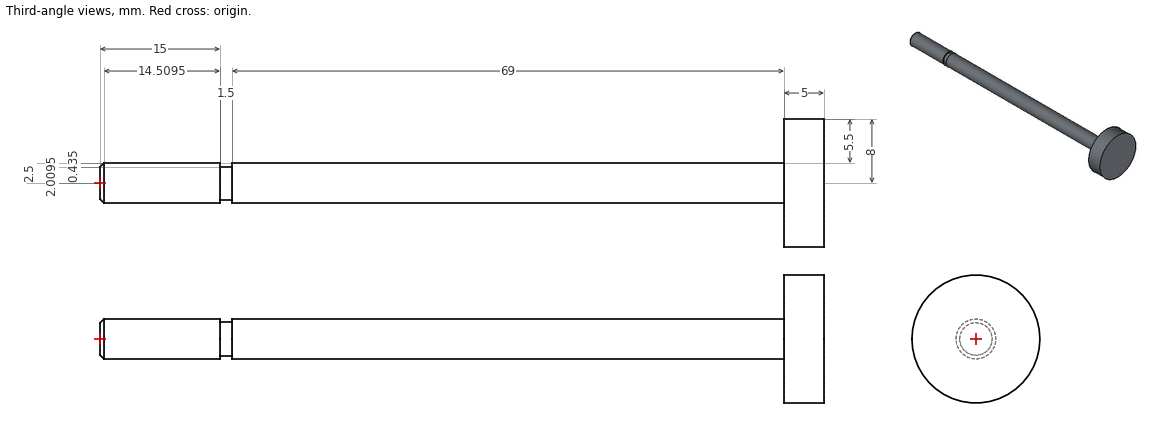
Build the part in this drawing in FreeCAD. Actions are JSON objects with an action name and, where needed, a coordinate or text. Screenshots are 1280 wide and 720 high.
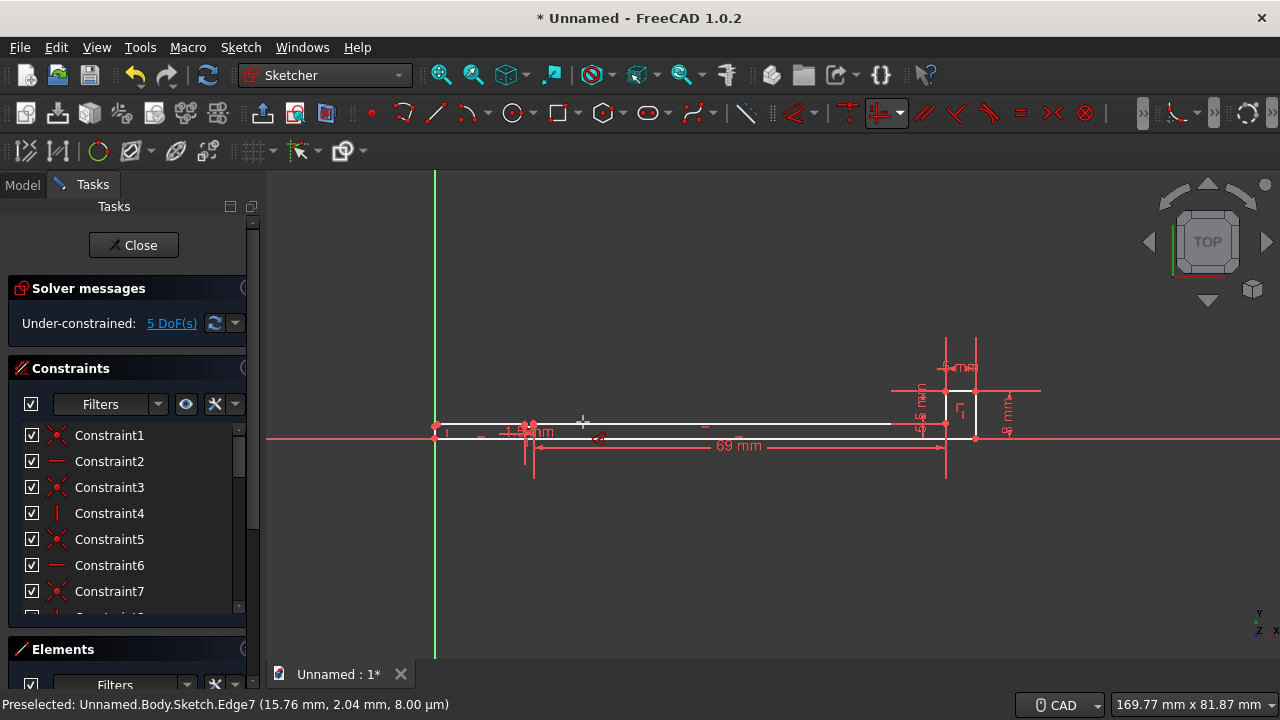
{"action": "scroll", "coordinate": [525, 427], "scroll_direction": "up", "scroll_amount": 8}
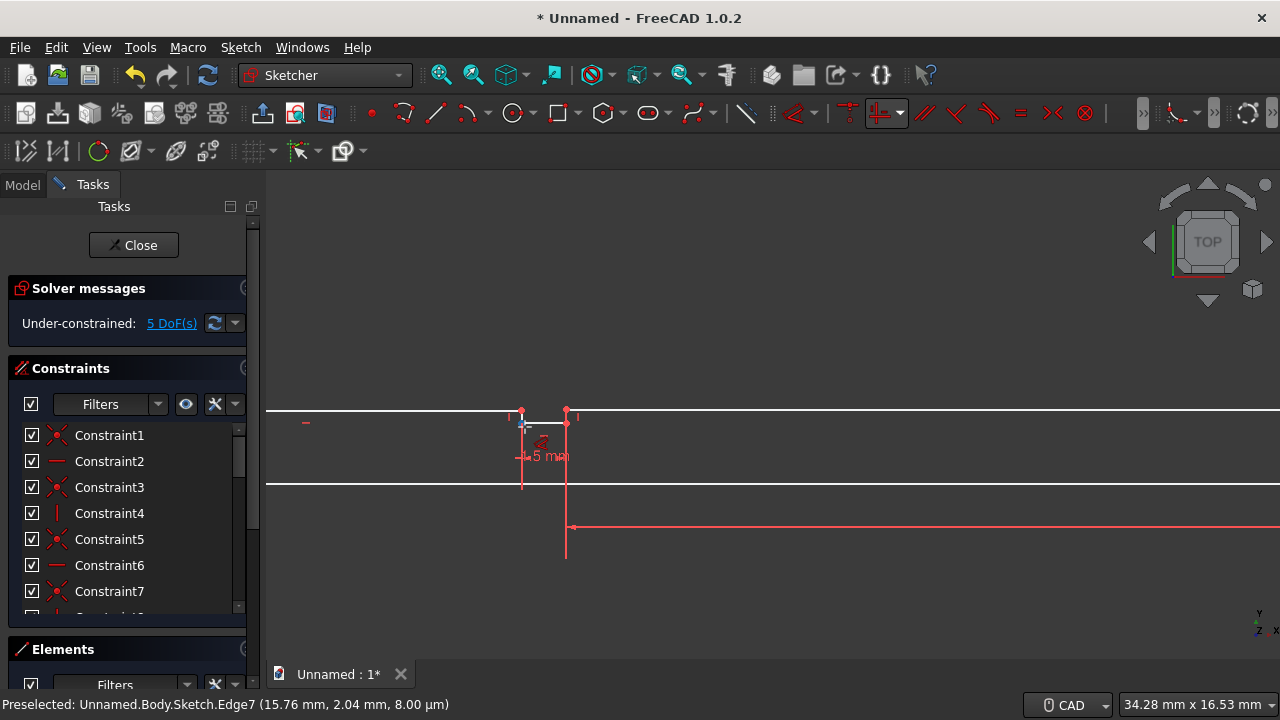
{"action": "left_click", "coordinate": [522, 423]}
{"action": "left_click", "coordinate": [408, 518]}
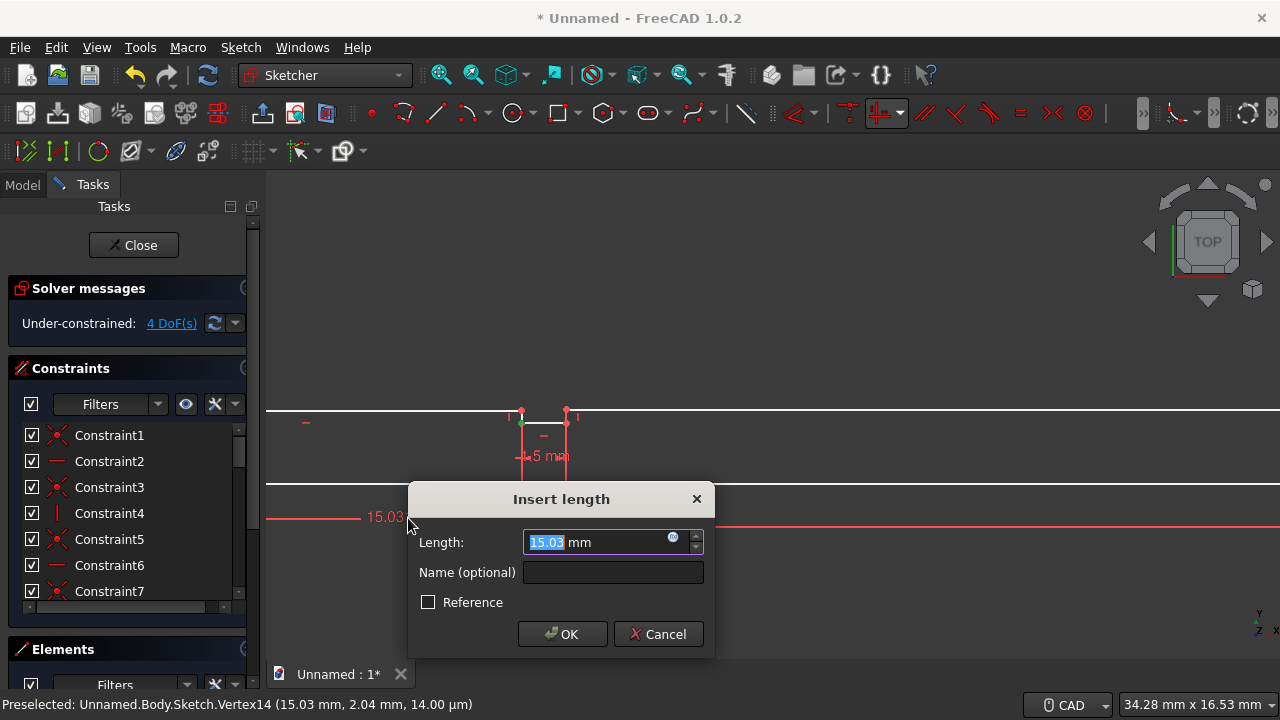
{"action": "type", "text": "15"}
{"action": "key", "text": "Return"}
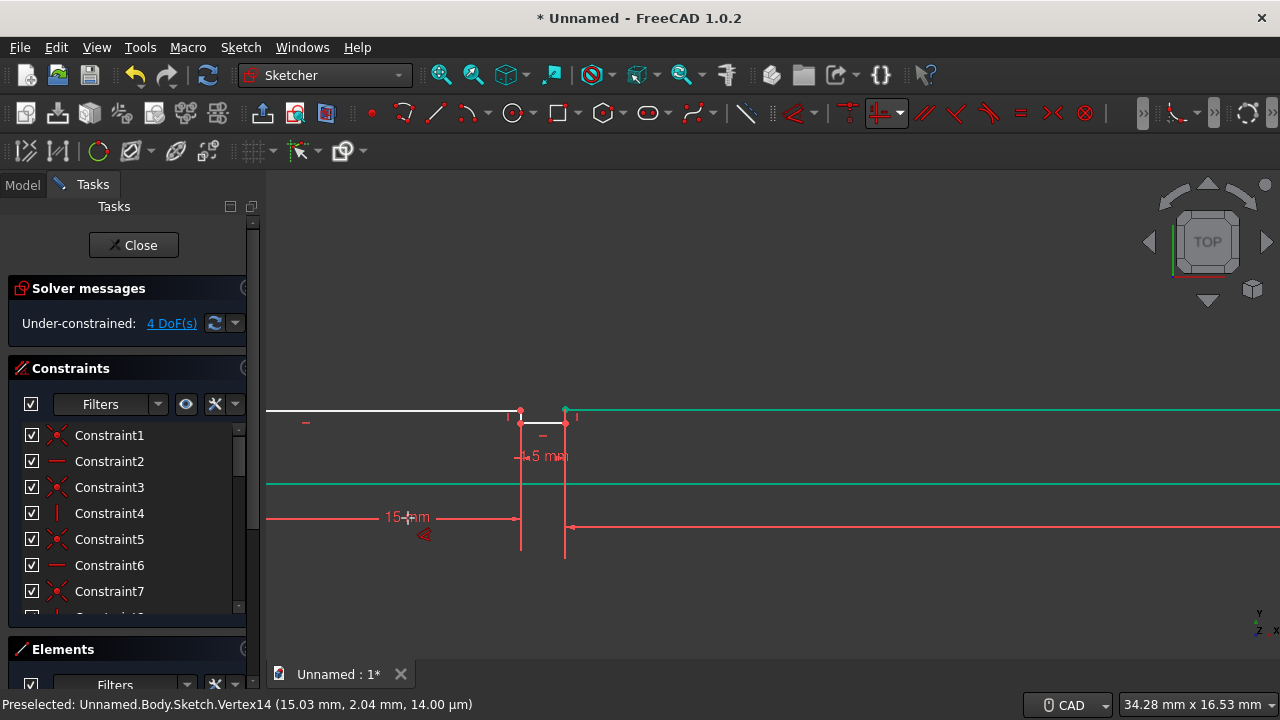
{"action": "left_click", "coordinate": [521, 411]}
{"action": "left_click", "coordinate": [579, 430]}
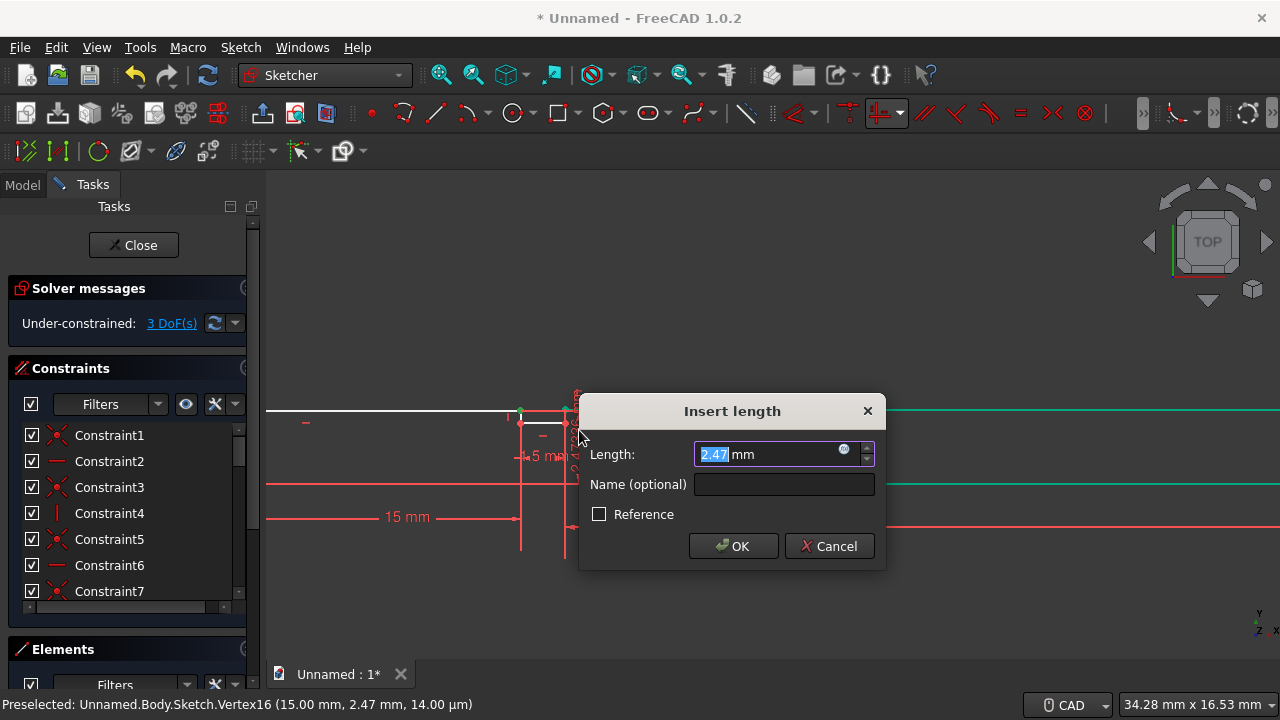
{"action": "type", "text": "2.5"}
{"action": "key", "text": "Return"}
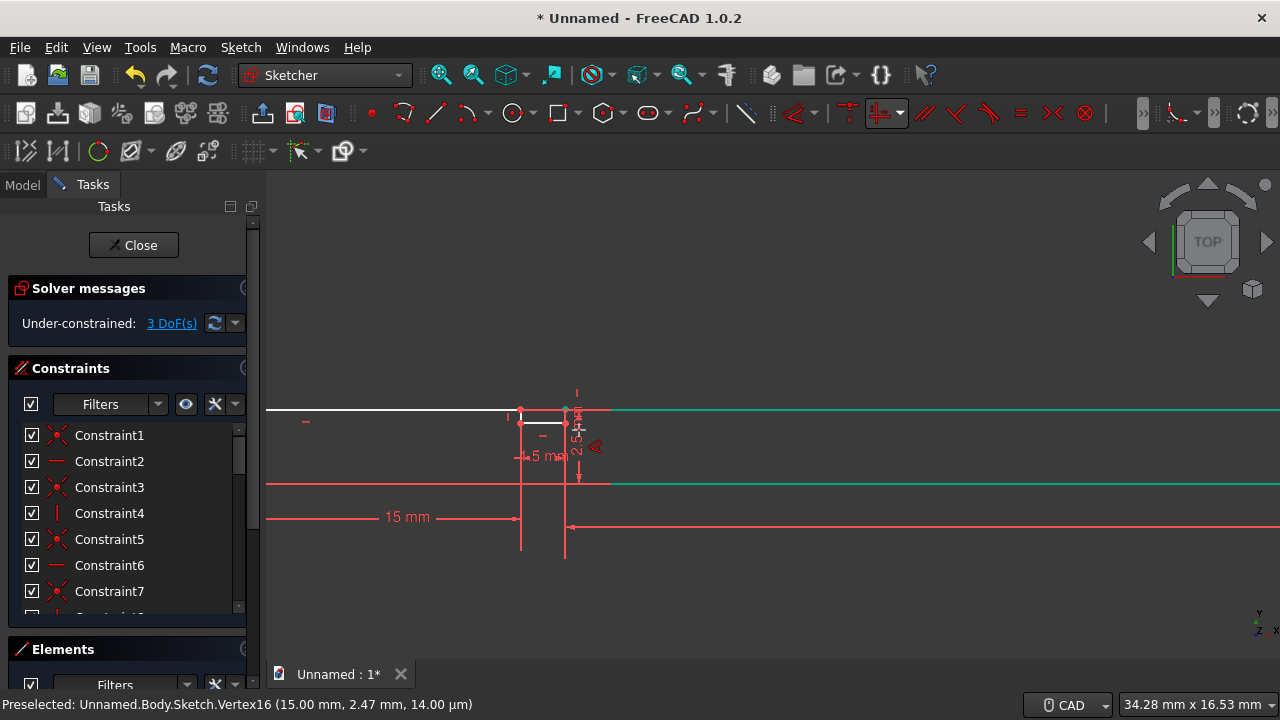
{"action": "scroll", "coordinate": [565, 417], "scroll_direction": "up", "scroll_amount": 6}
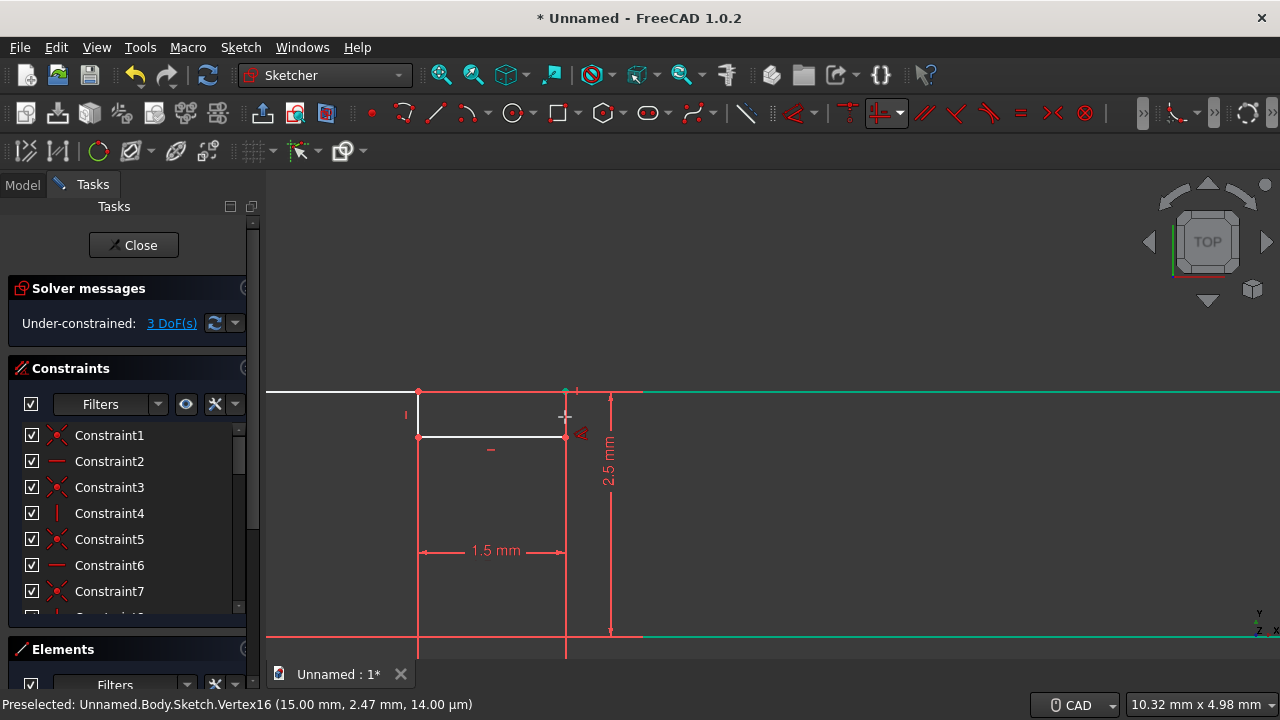
{"action": "left_click", "coordinate": [566, 415]}
{"action": "left_click", "coordinate": [532, 415]}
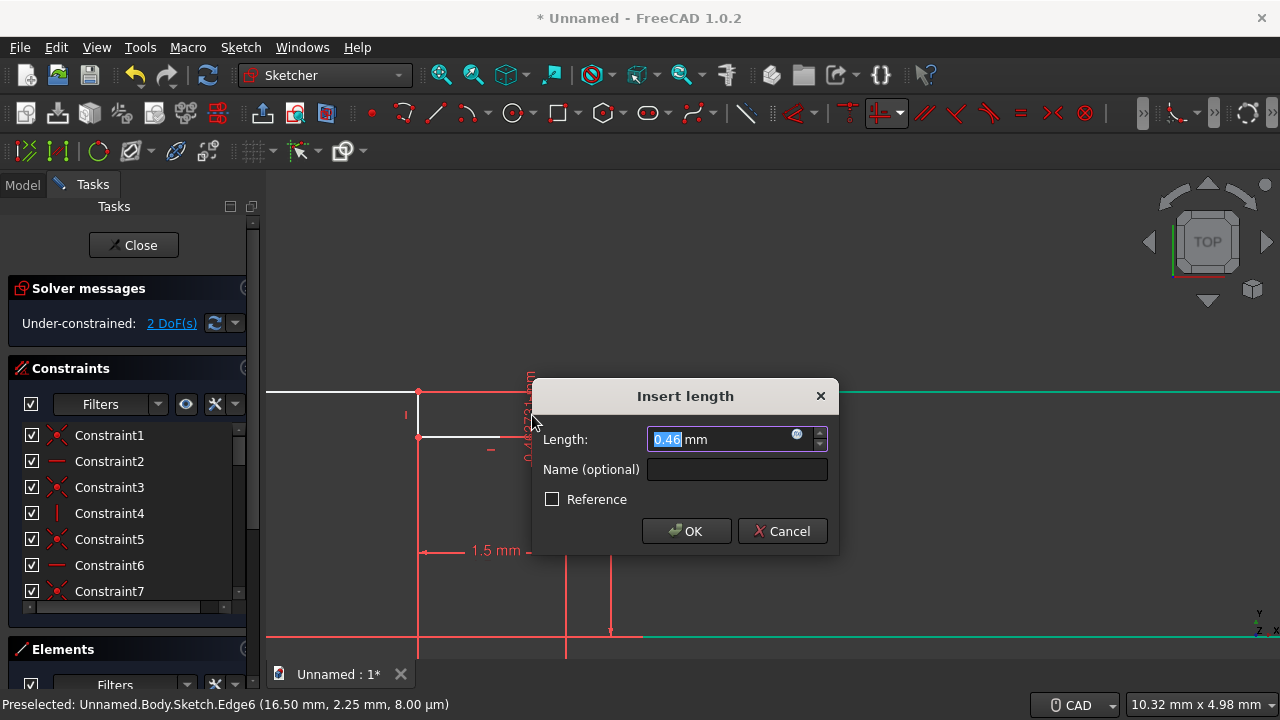
{"action": "type", "text": "0.435"}
{"action": "key", "text": "Return"}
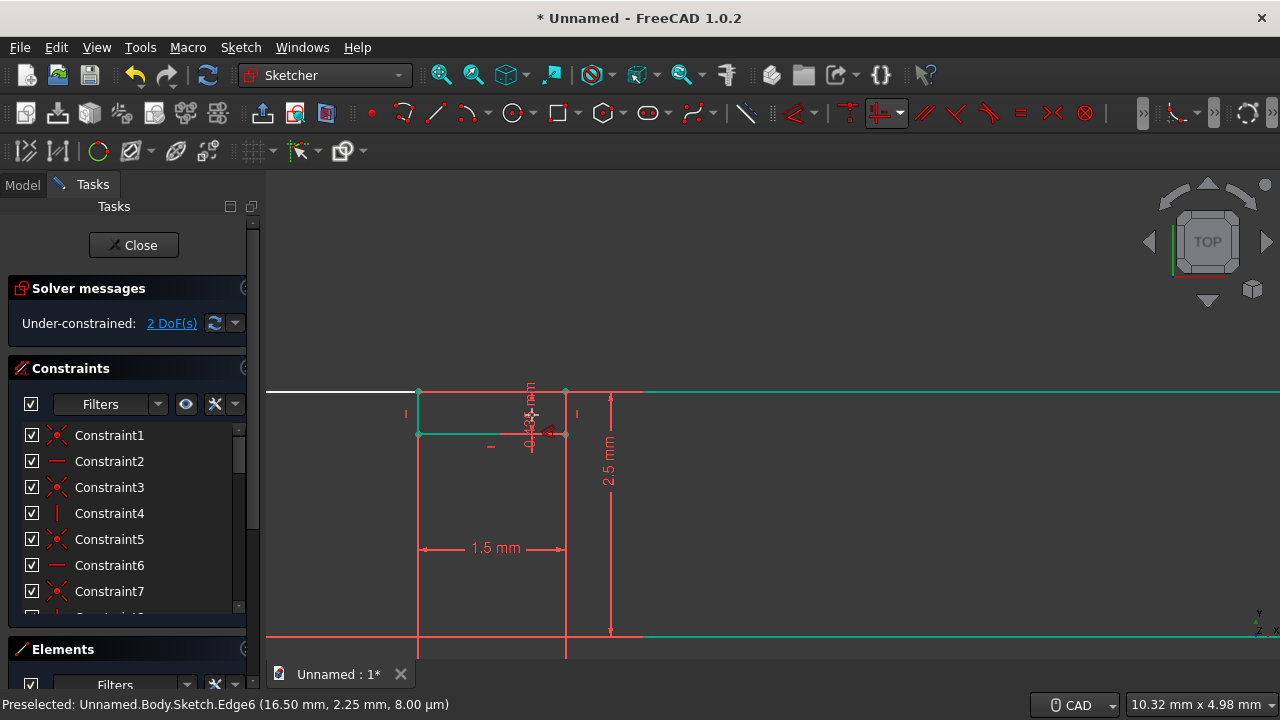
{"action": "scroll", "coordinate": [531, 426], "scroll_direction": "down", "scroll_amount": 14}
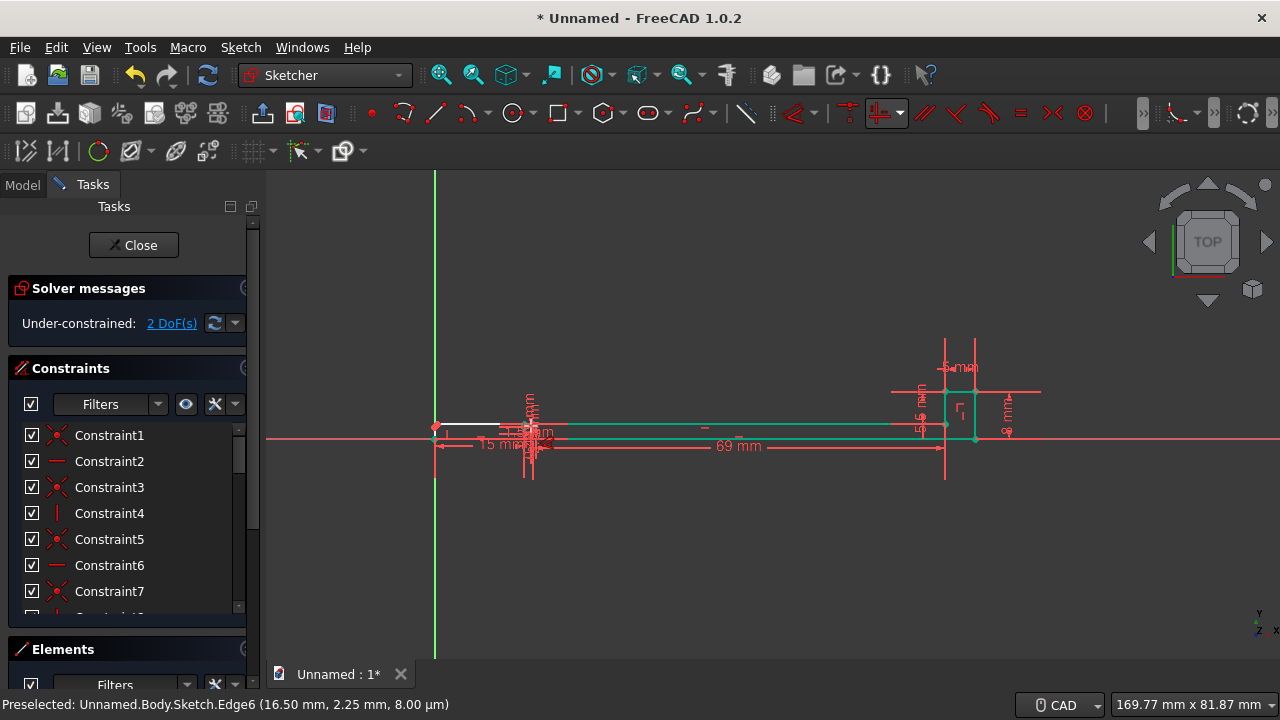
{"action": "scroll", "coordinate": [435, 431], "scroll_direction": "up", "scroll_amount": 7}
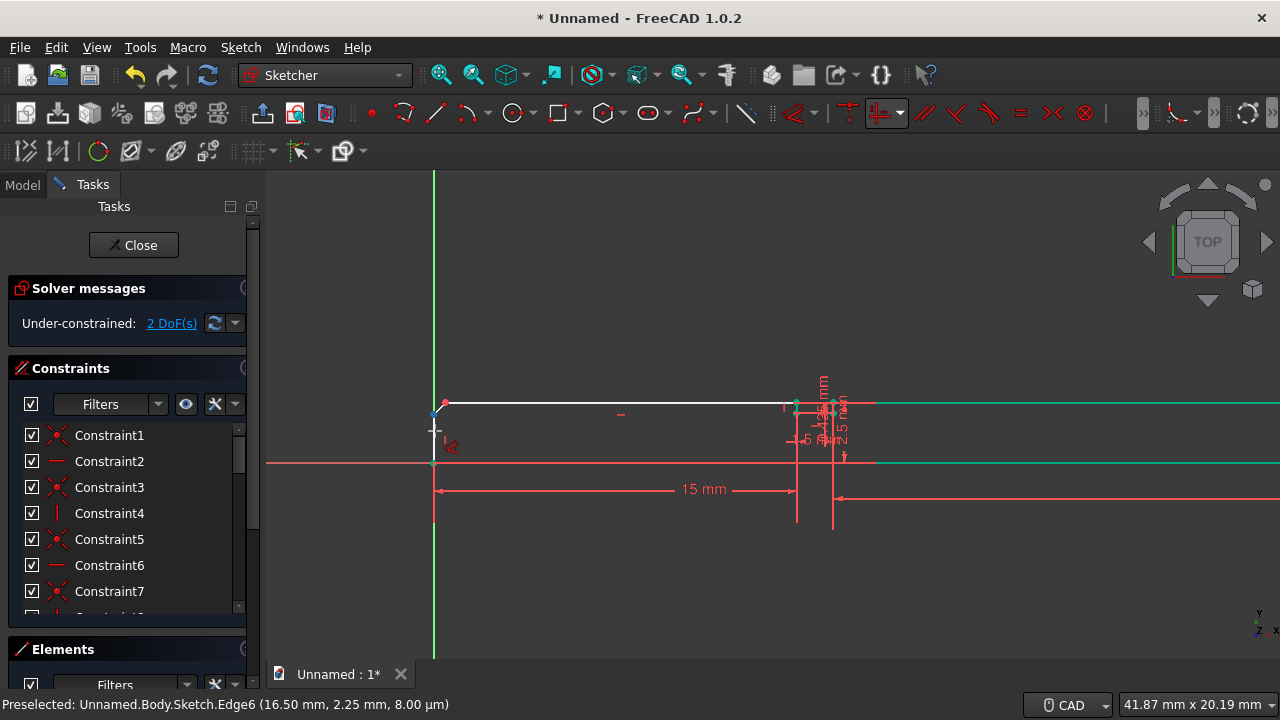
{"action": "left_click", "coordinate": [434, 429]}
{"action": "left_click", "coordinate": [400, 439]}